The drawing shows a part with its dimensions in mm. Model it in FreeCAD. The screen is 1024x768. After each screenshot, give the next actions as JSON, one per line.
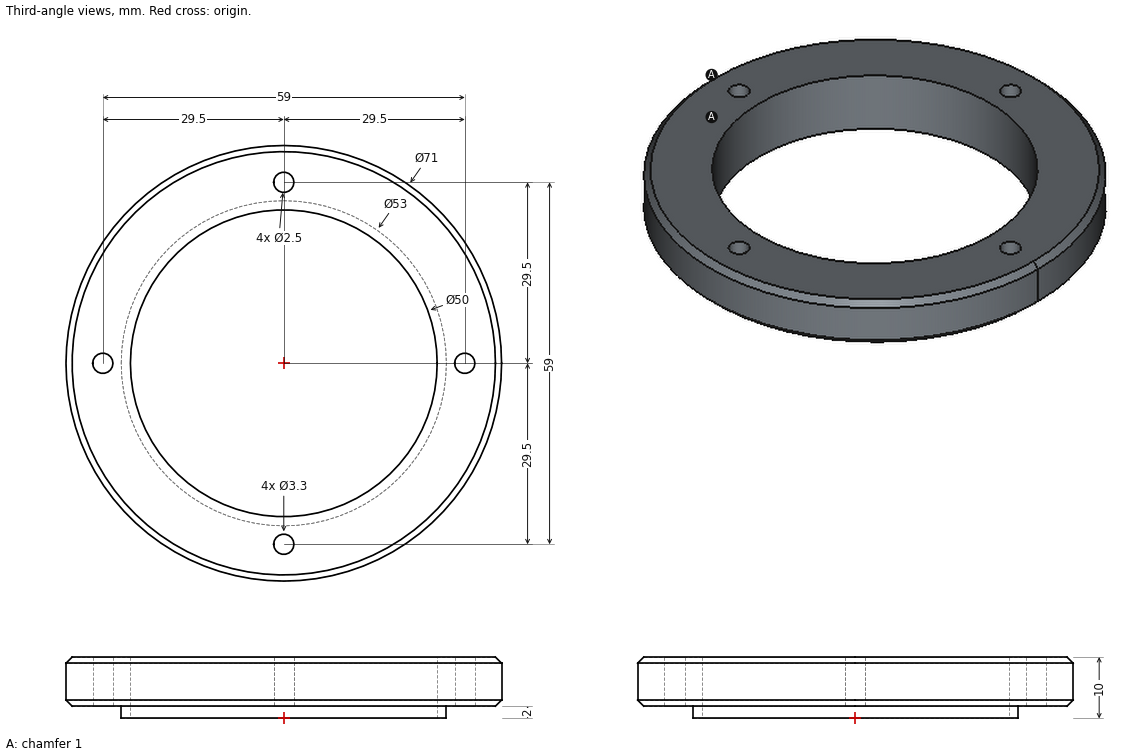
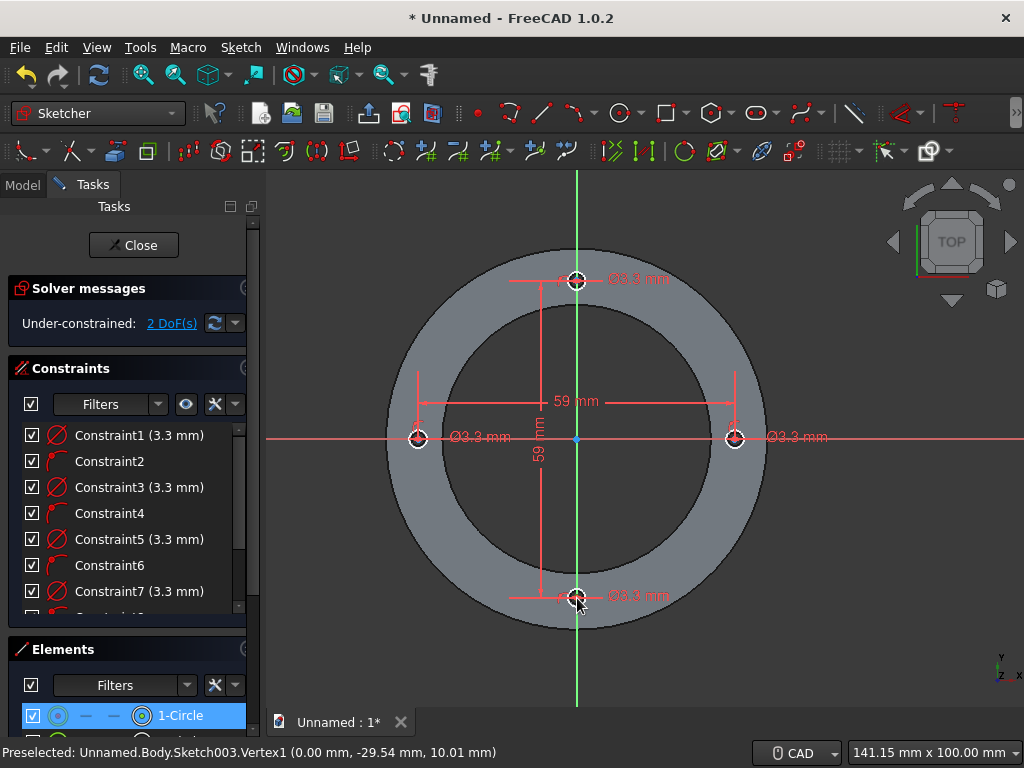
{"action": "key", "text": "i"}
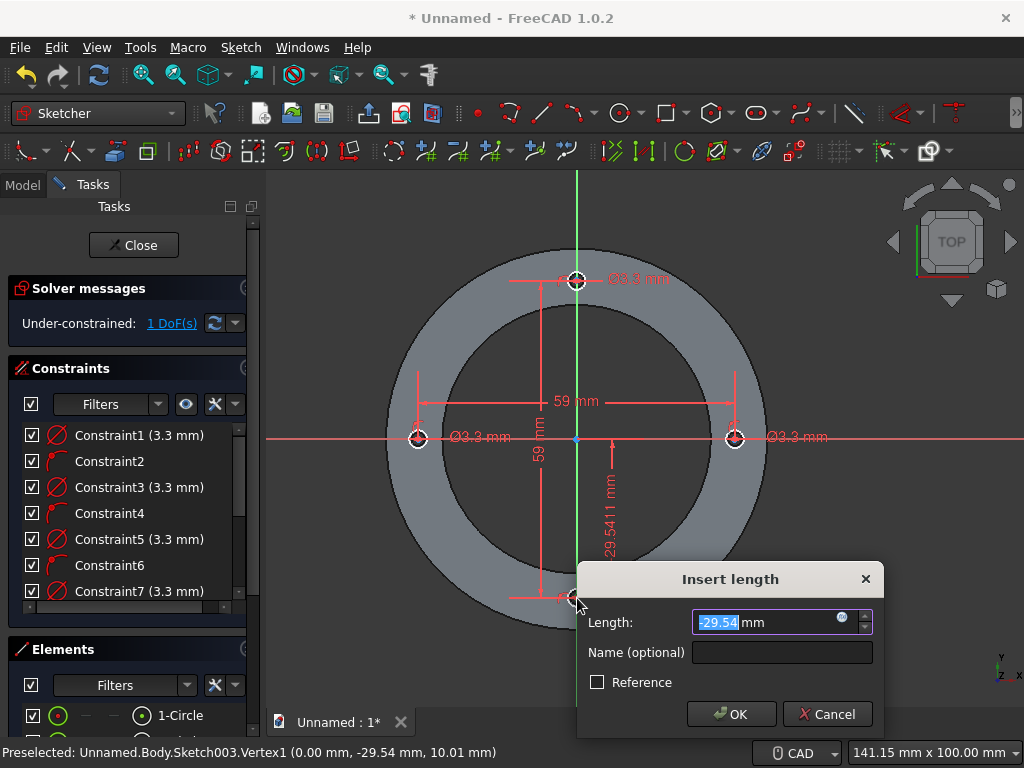
{"action": "type", "text": "-29.5"}
{"action": "key", "text": "Return"}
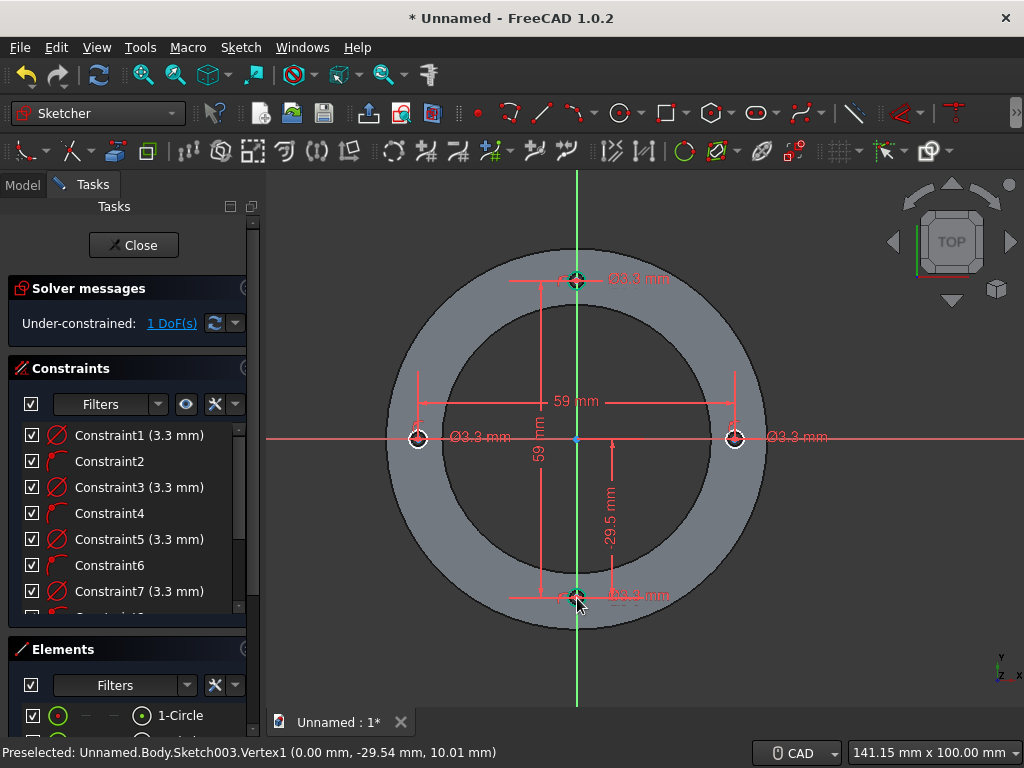
{"action": "left_click", "coordinate": [418, 439]}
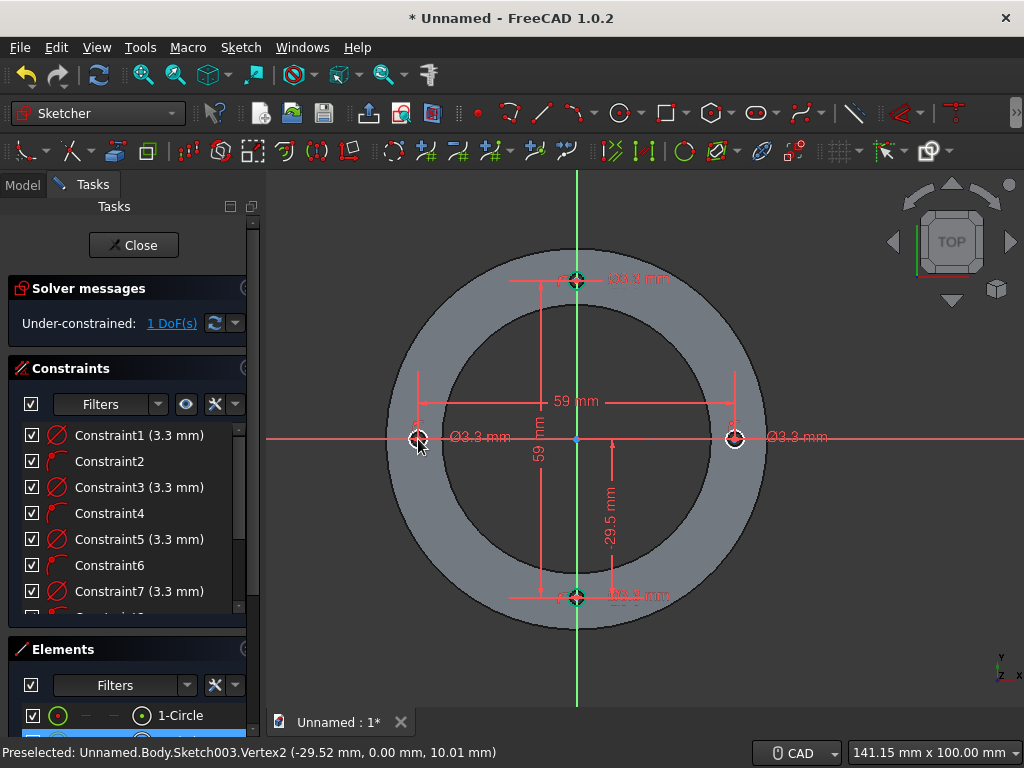
{"action": "key", "text": "l"}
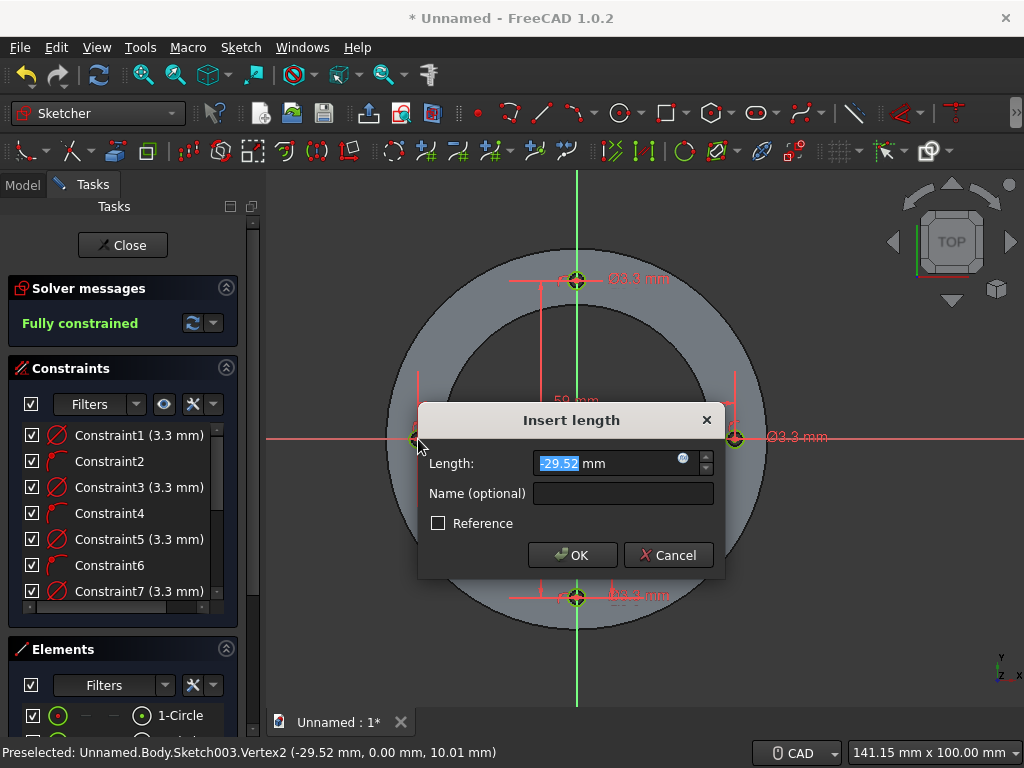
{"action": "type", "text": "-29.5"}
{"action": "key", "text": "Return"}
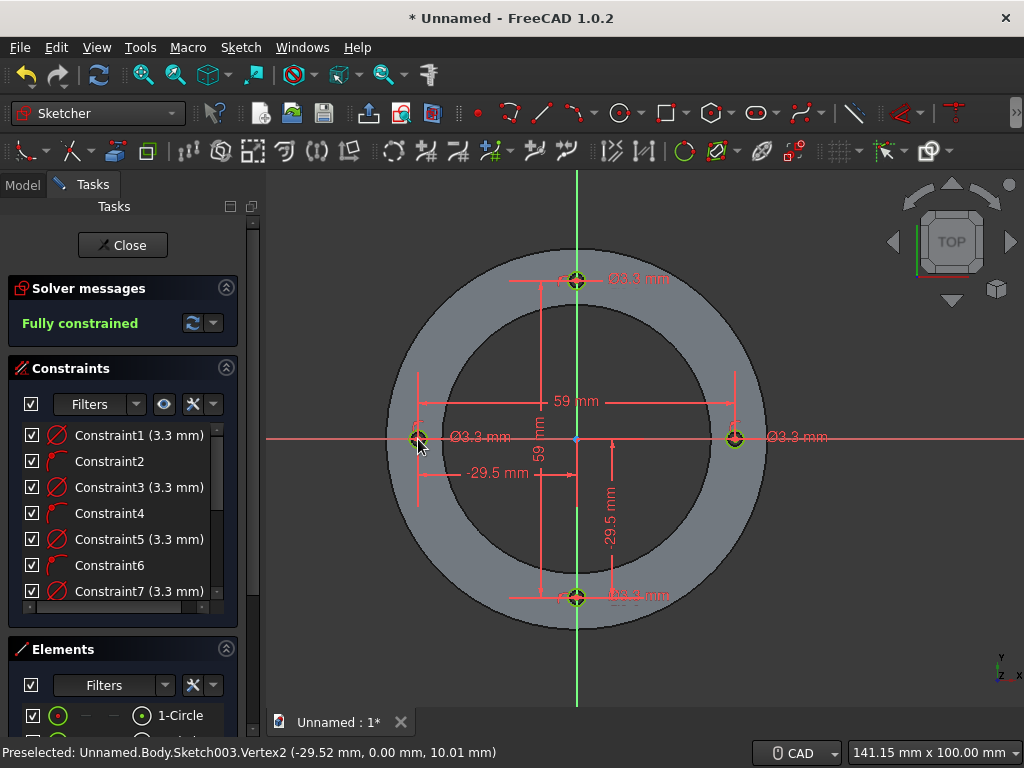
{"action": "left_click", "coordinate": [123, 245]}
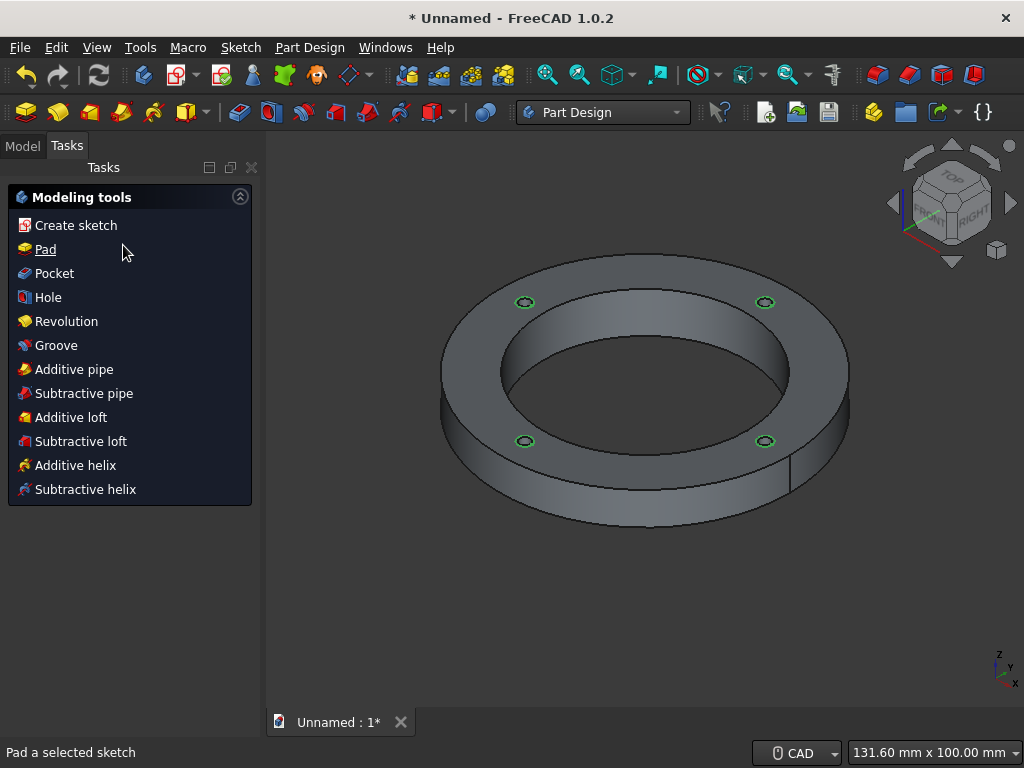
{"action": "left_click", "coordinate": [240, 112]}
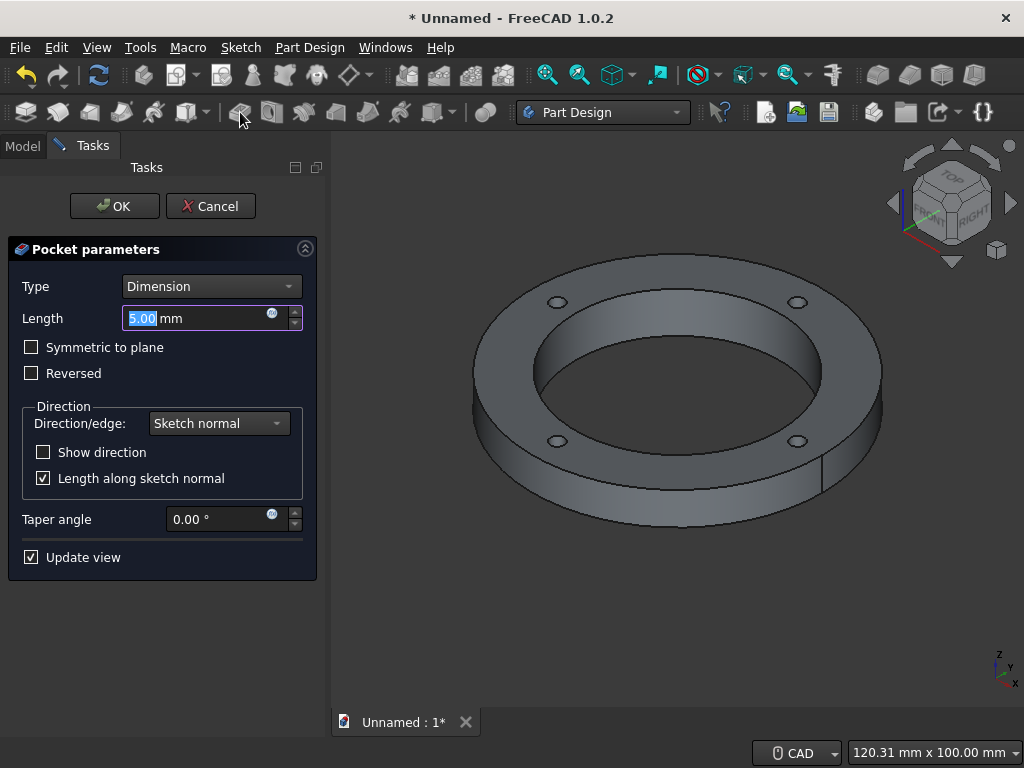
{"action": "left_click", "coordinate": [212, 286]}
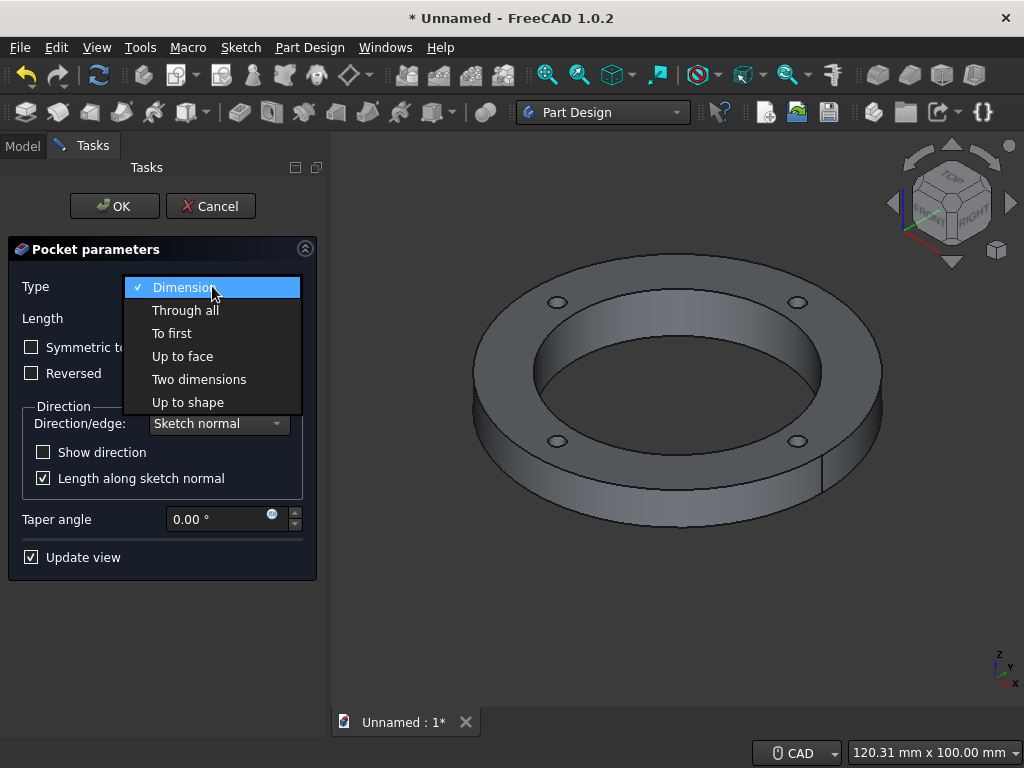
{"action": "left_click", "coordinate": [212, 310]}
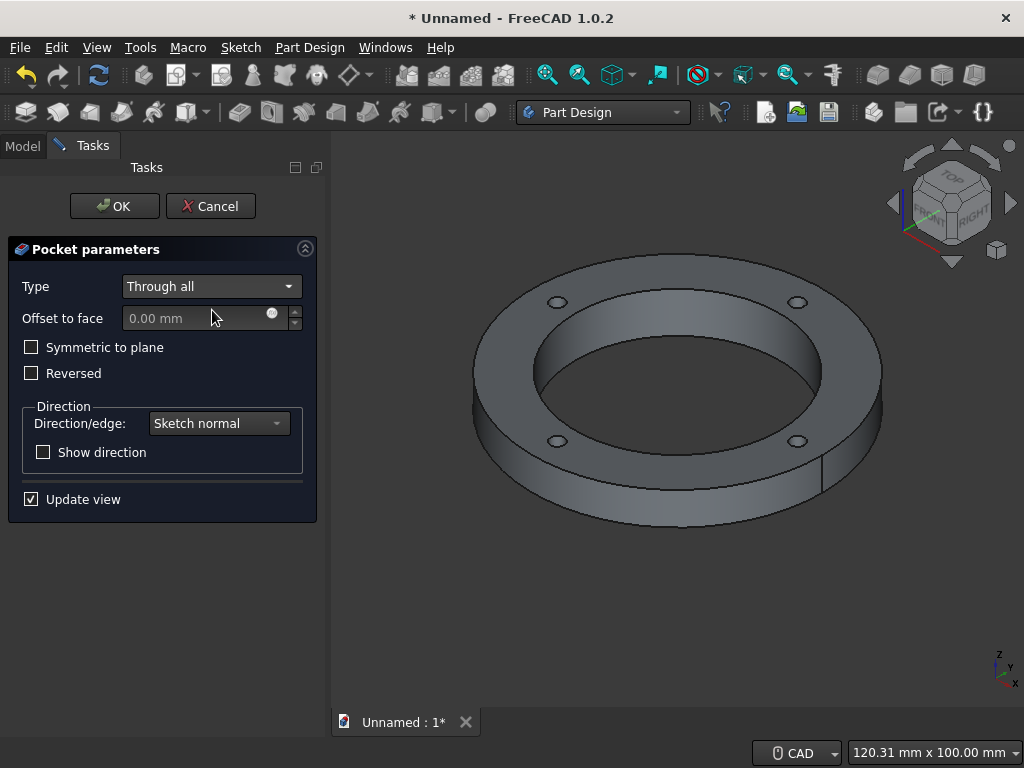
{"action": "left_click", "coordinate": [115, 206]}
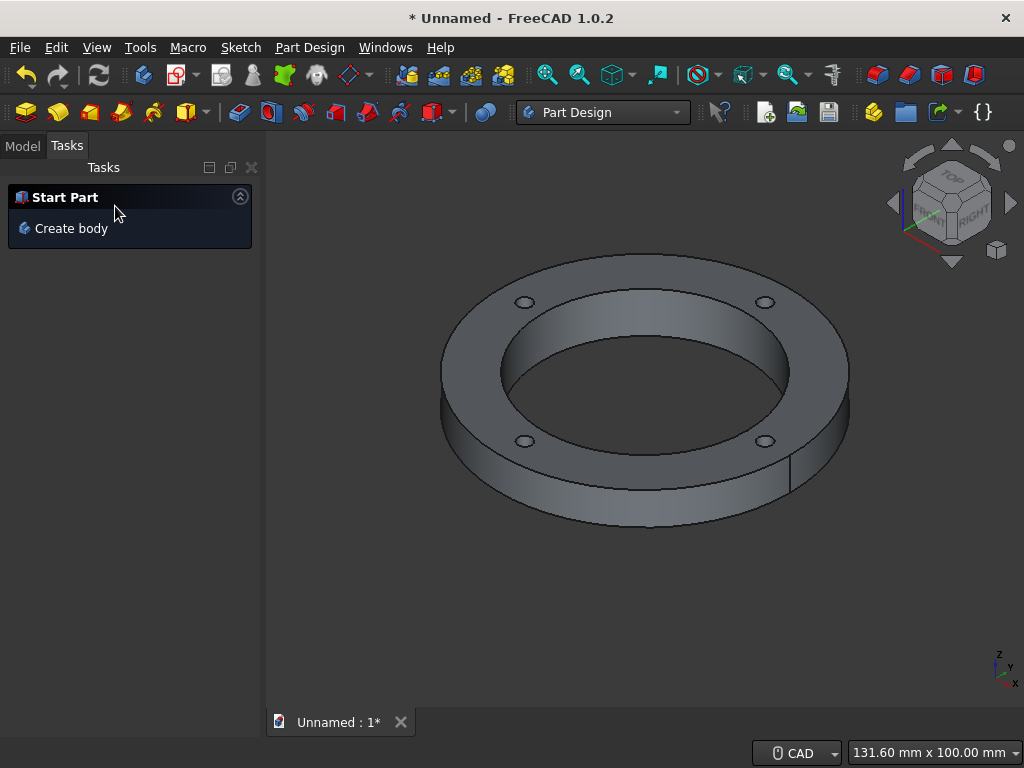
{"action": "left_click", "coordinate": [463, 425]}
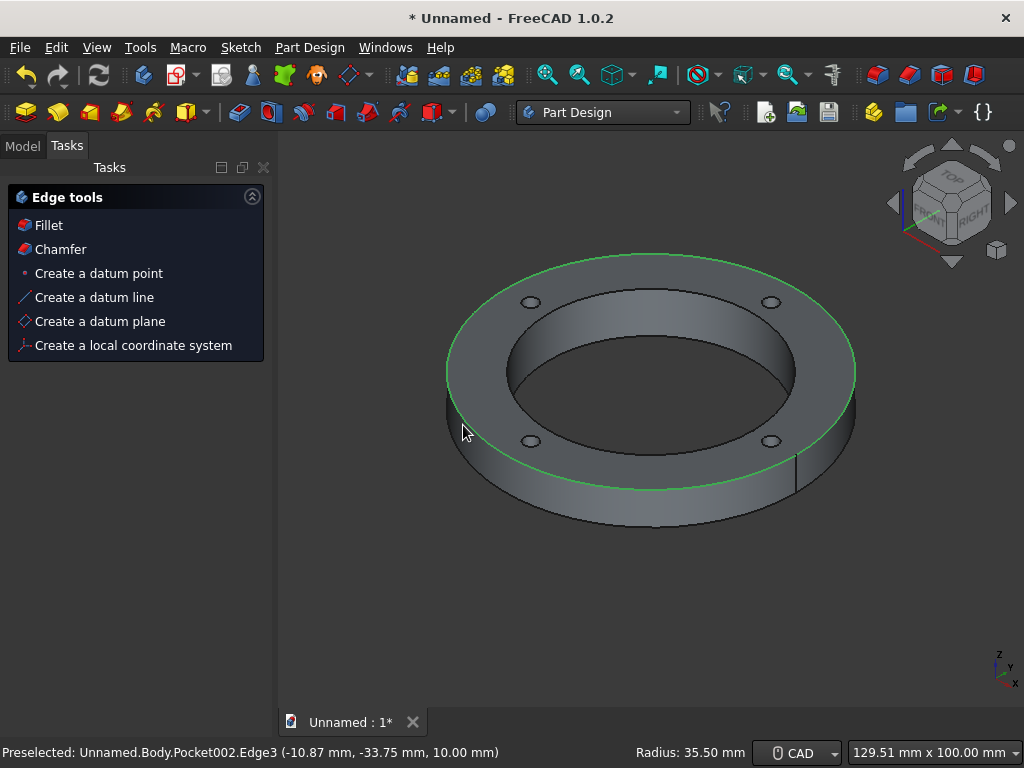
{"action": "key", "text": "2"}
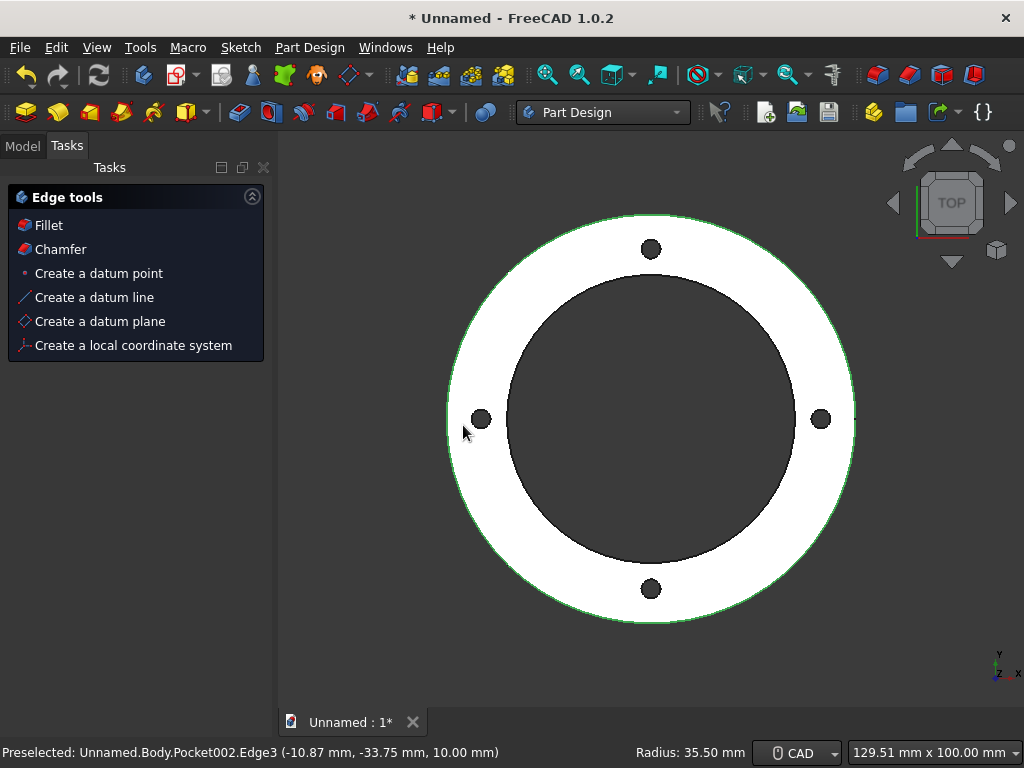
{"action": "key", "text": "0"}